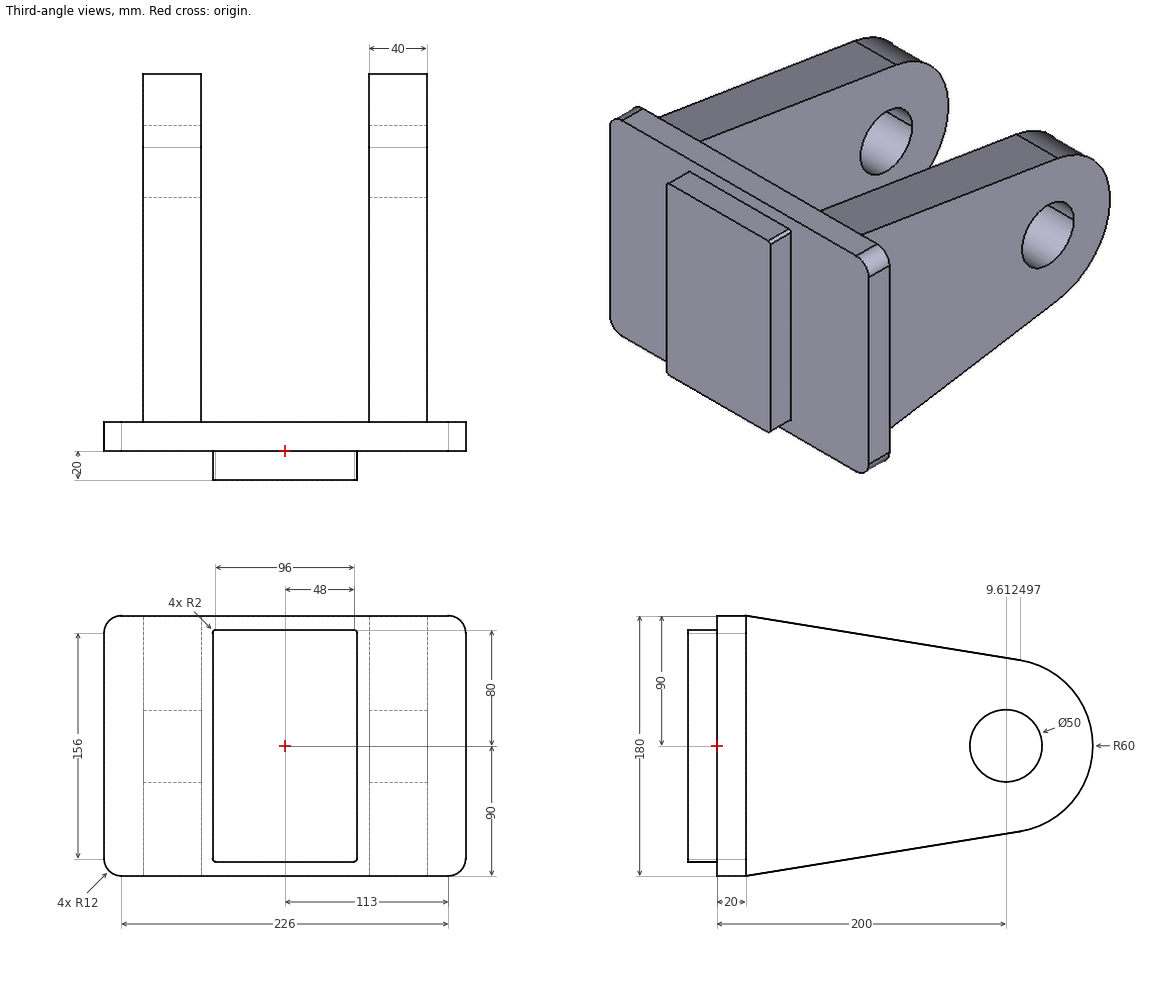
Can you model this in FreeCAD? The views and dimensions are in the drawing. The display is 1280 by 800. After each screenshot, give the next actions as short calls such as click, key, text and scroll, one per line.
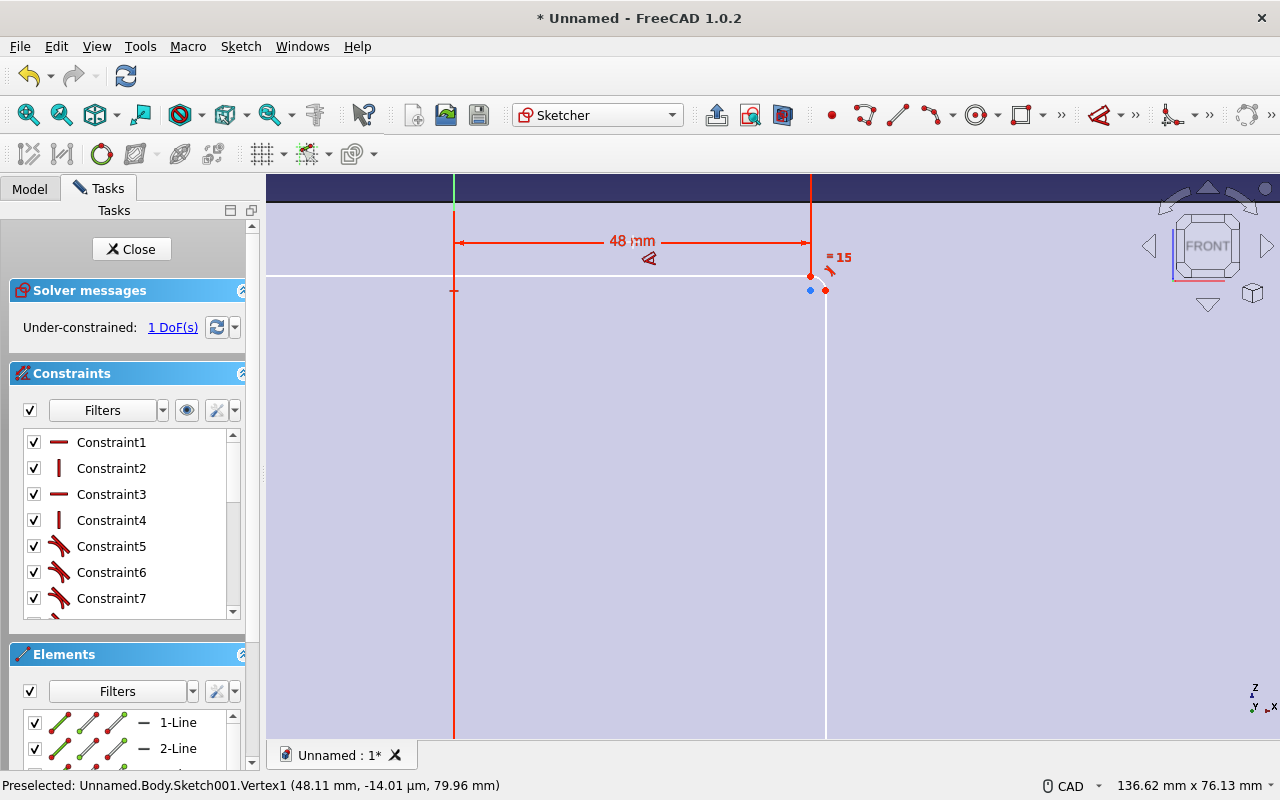
click(811, 276)
click(845, 494)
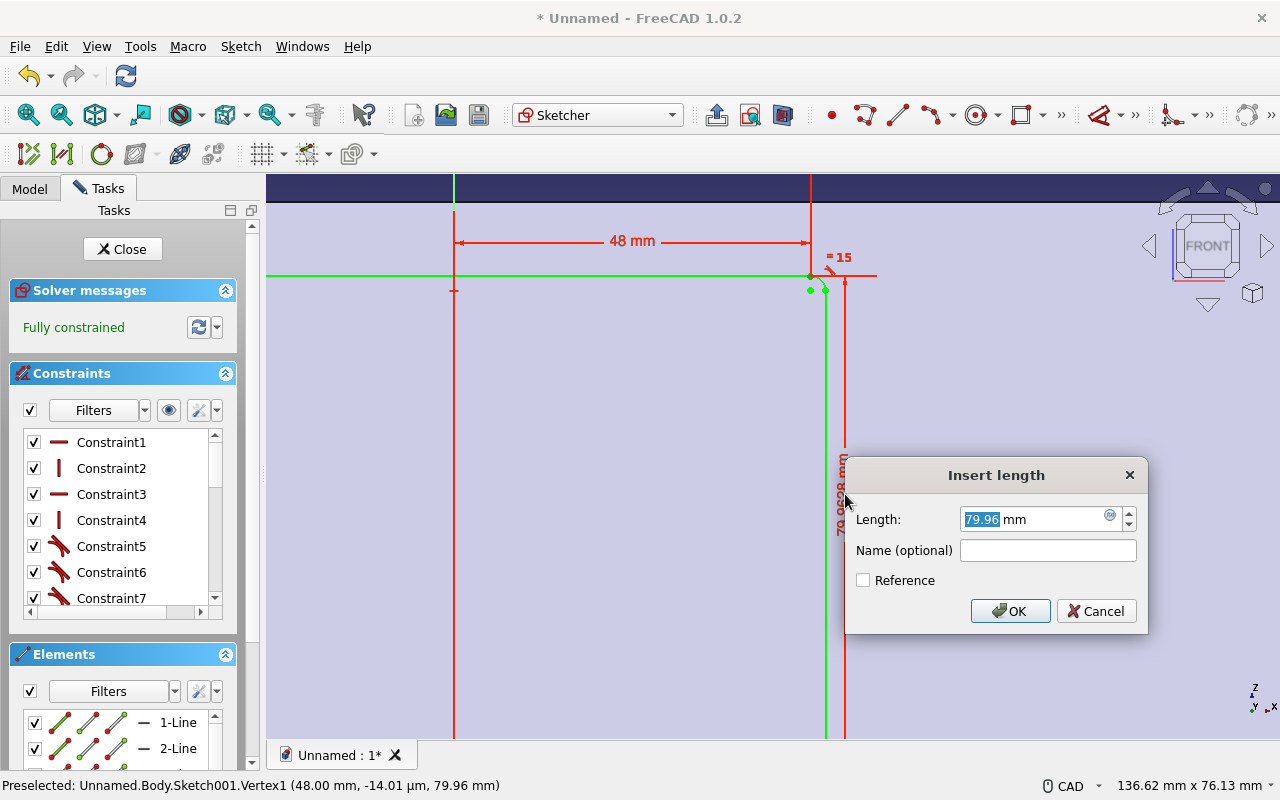
text(80)
key(Return)
key(Escape)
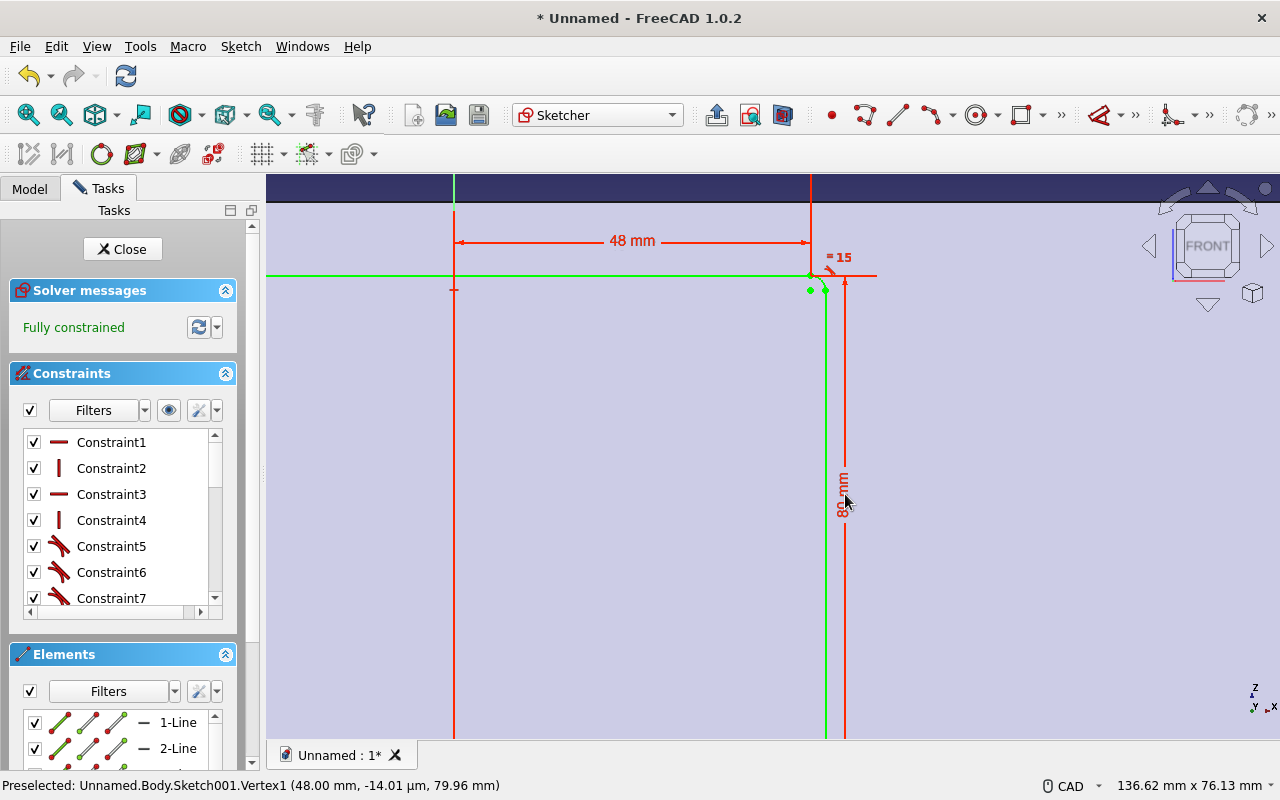
click(123, 249)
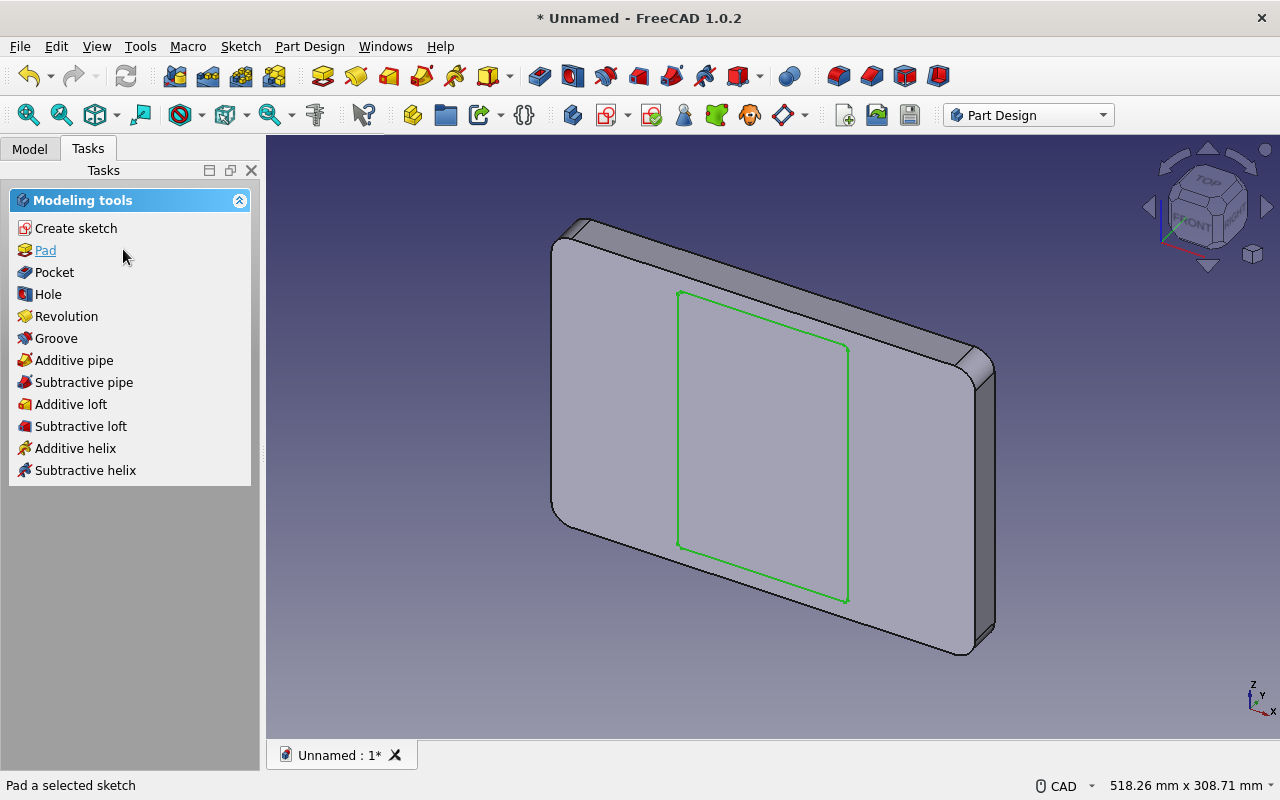
click(323, 76)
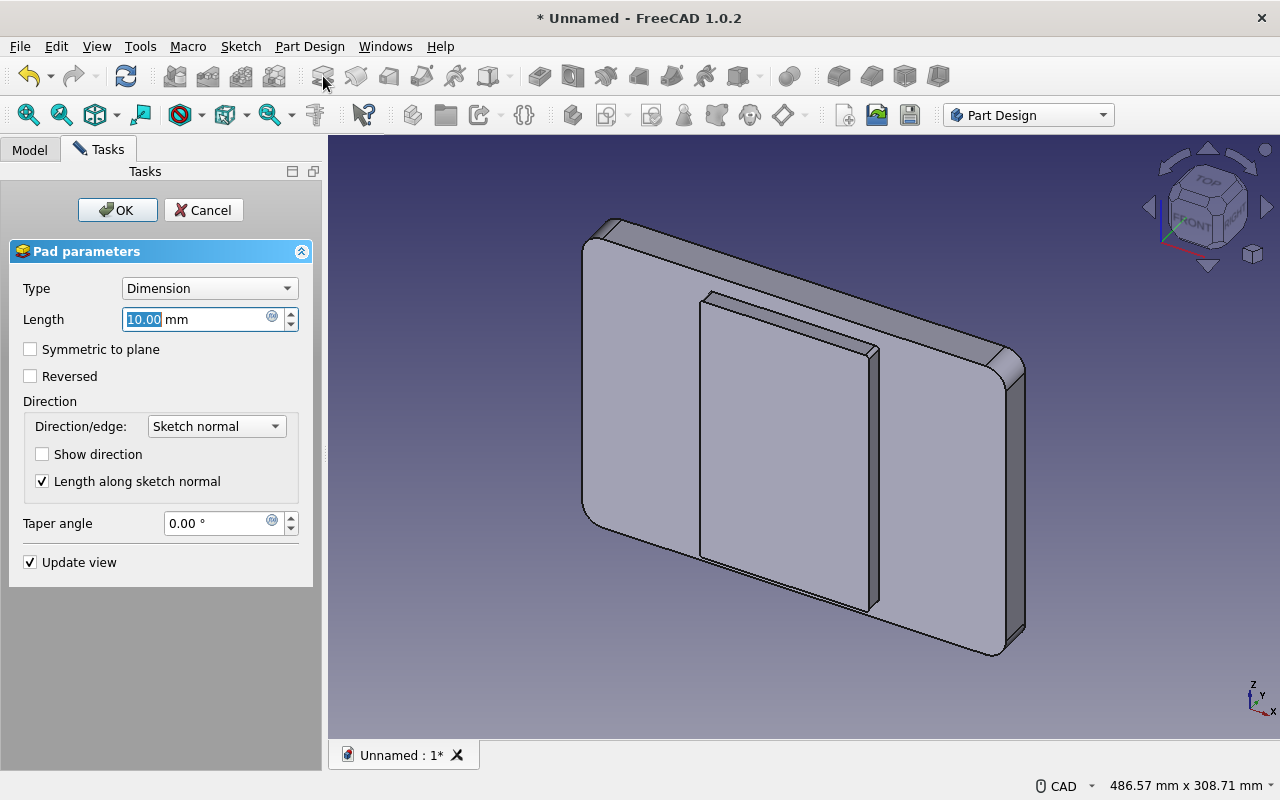
text(20)
key(Tab)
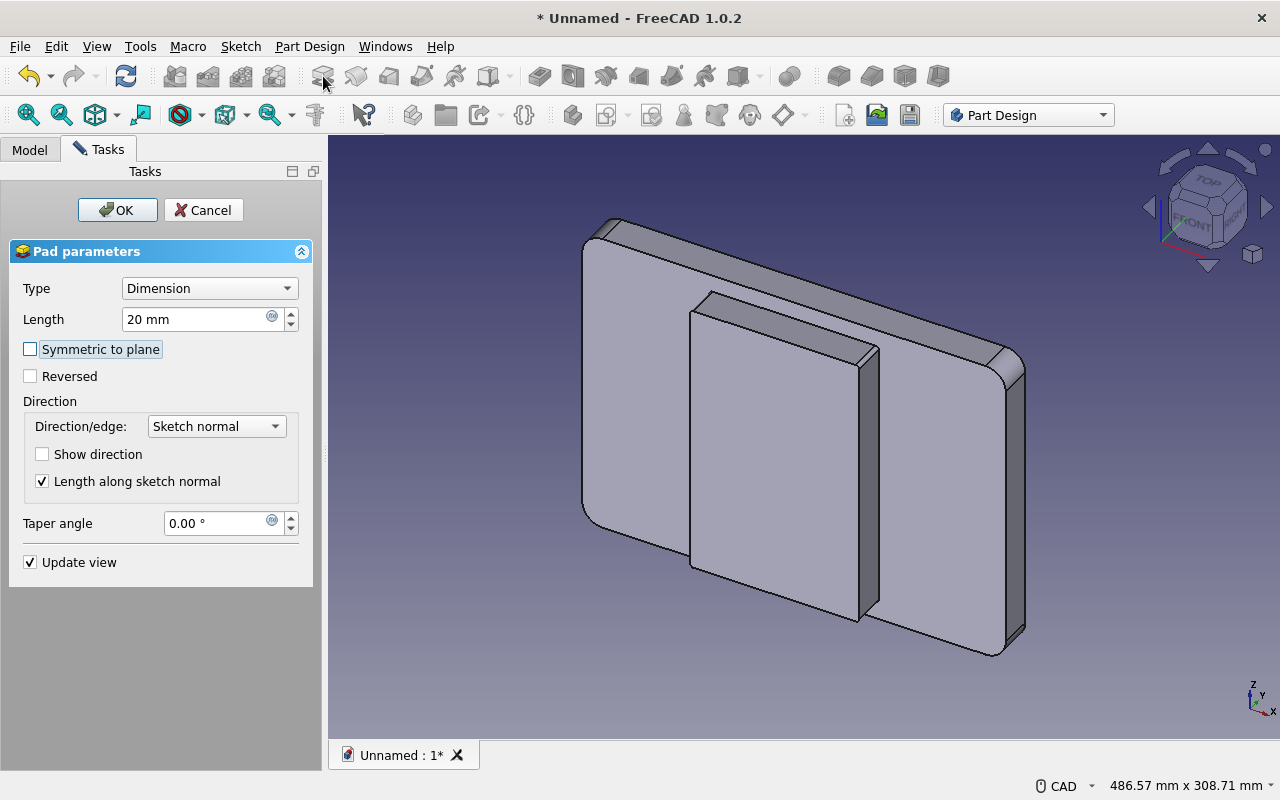
click(118, 210)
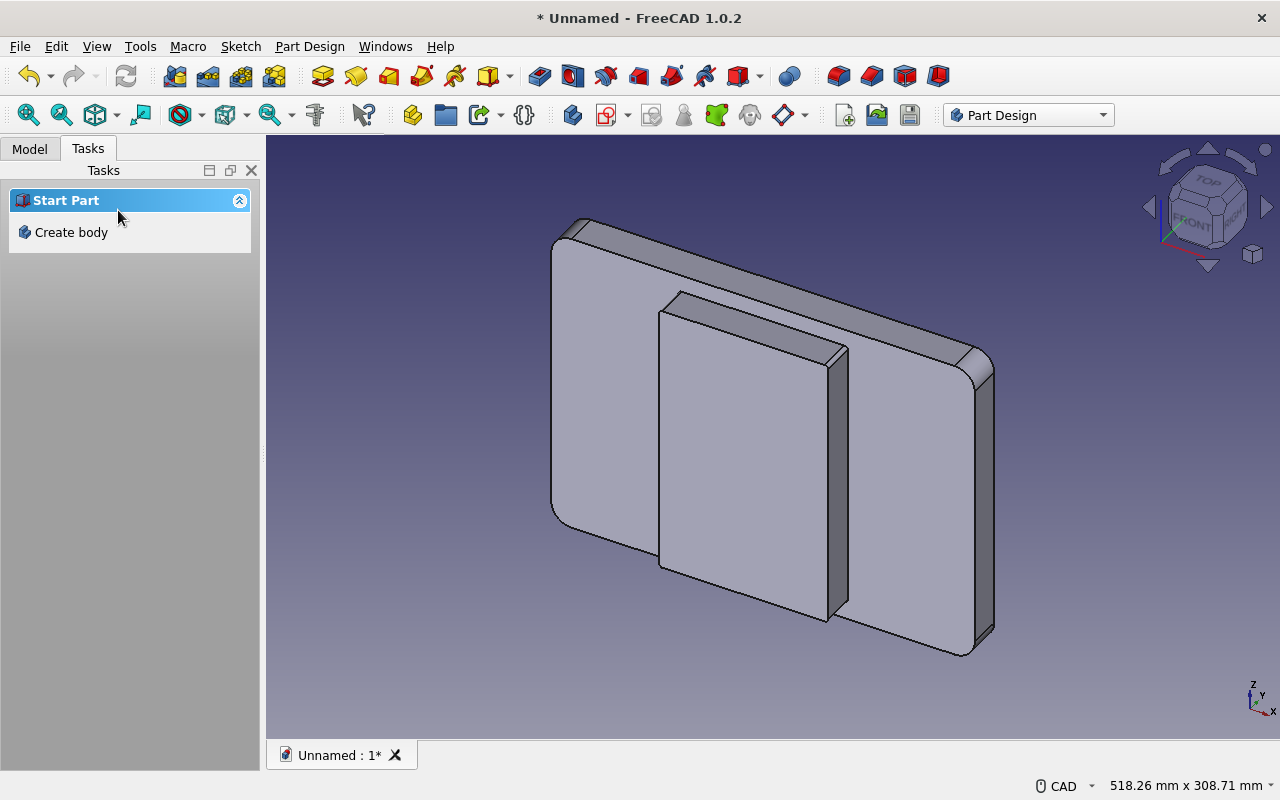
click(30, 148)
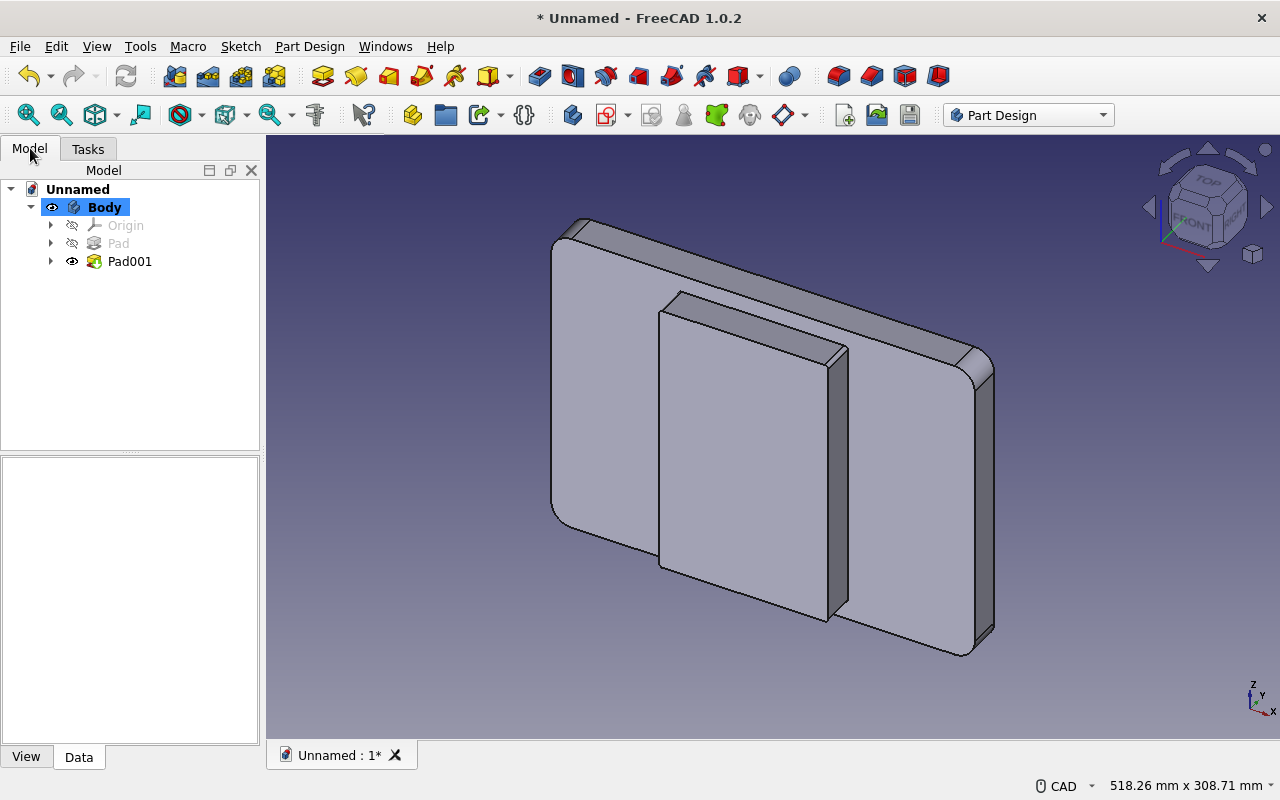
click(51, 225)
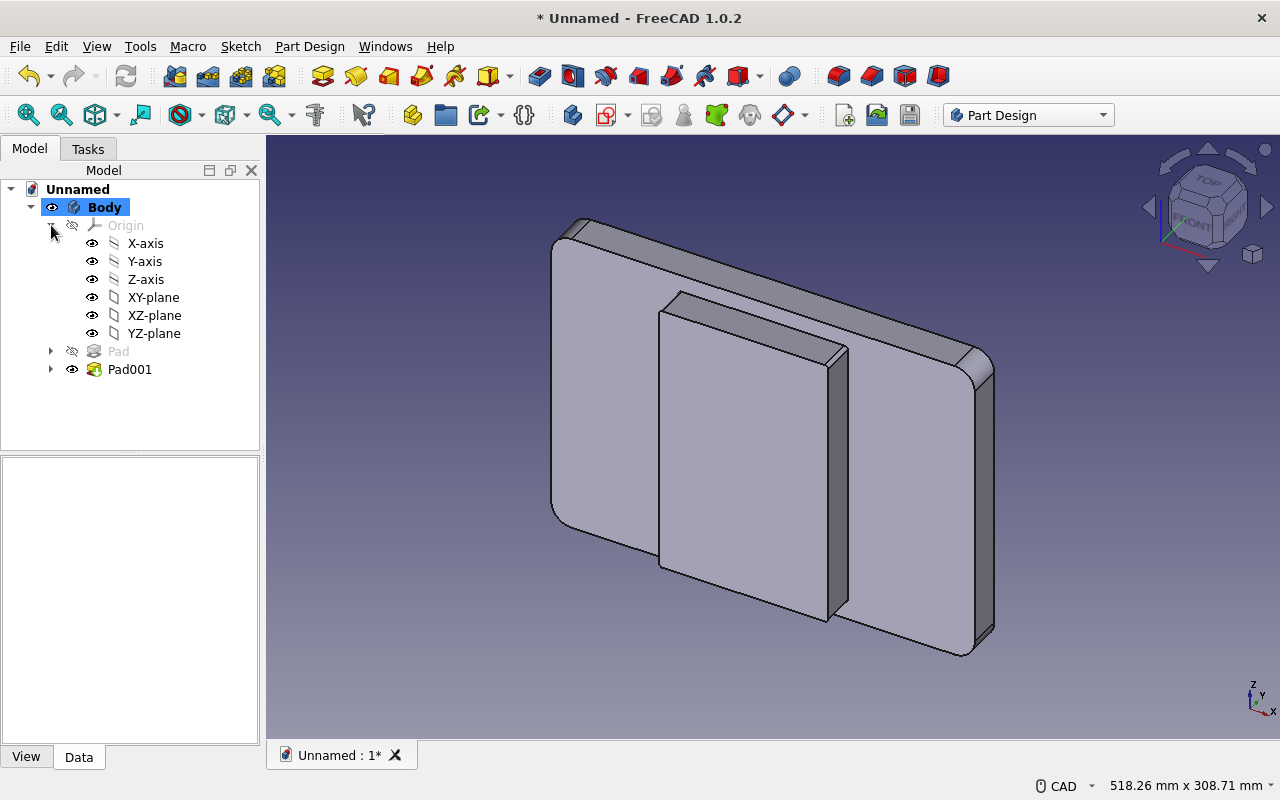
click(137, 333)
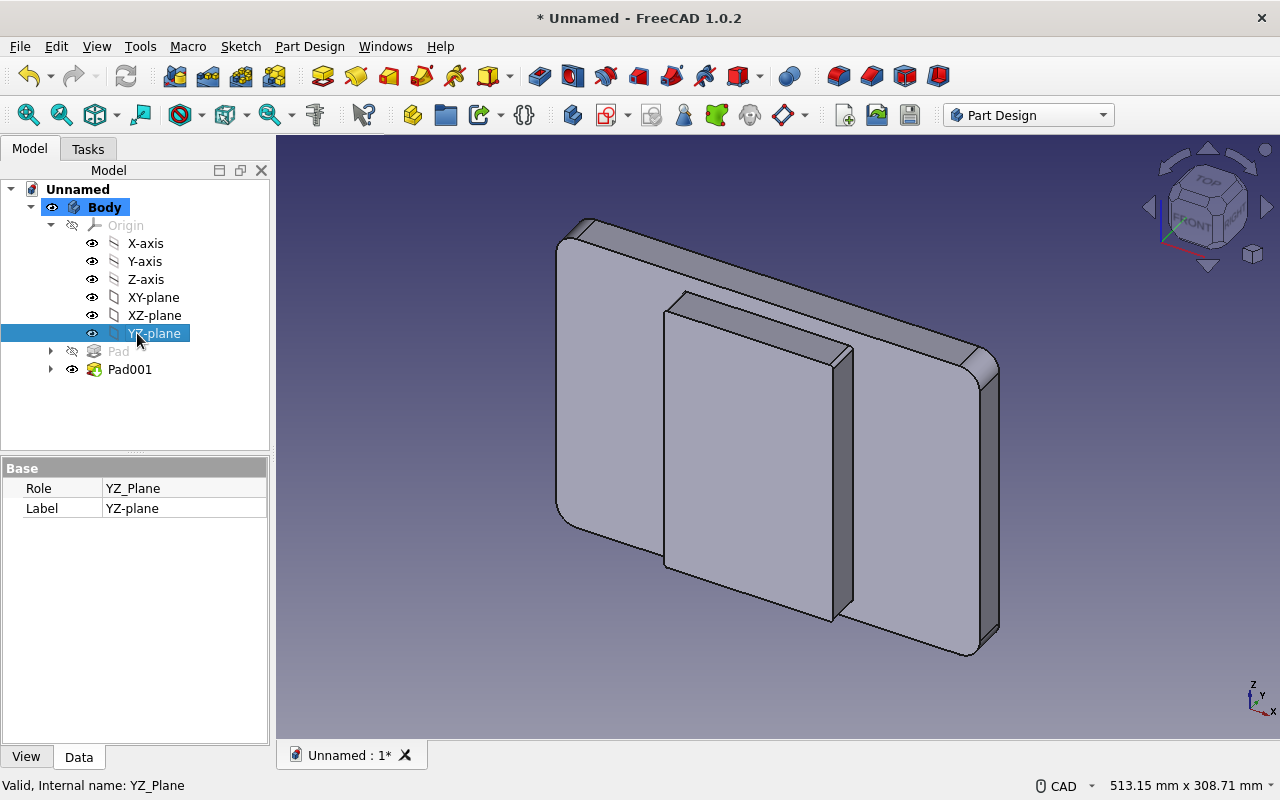
click(782, 116)